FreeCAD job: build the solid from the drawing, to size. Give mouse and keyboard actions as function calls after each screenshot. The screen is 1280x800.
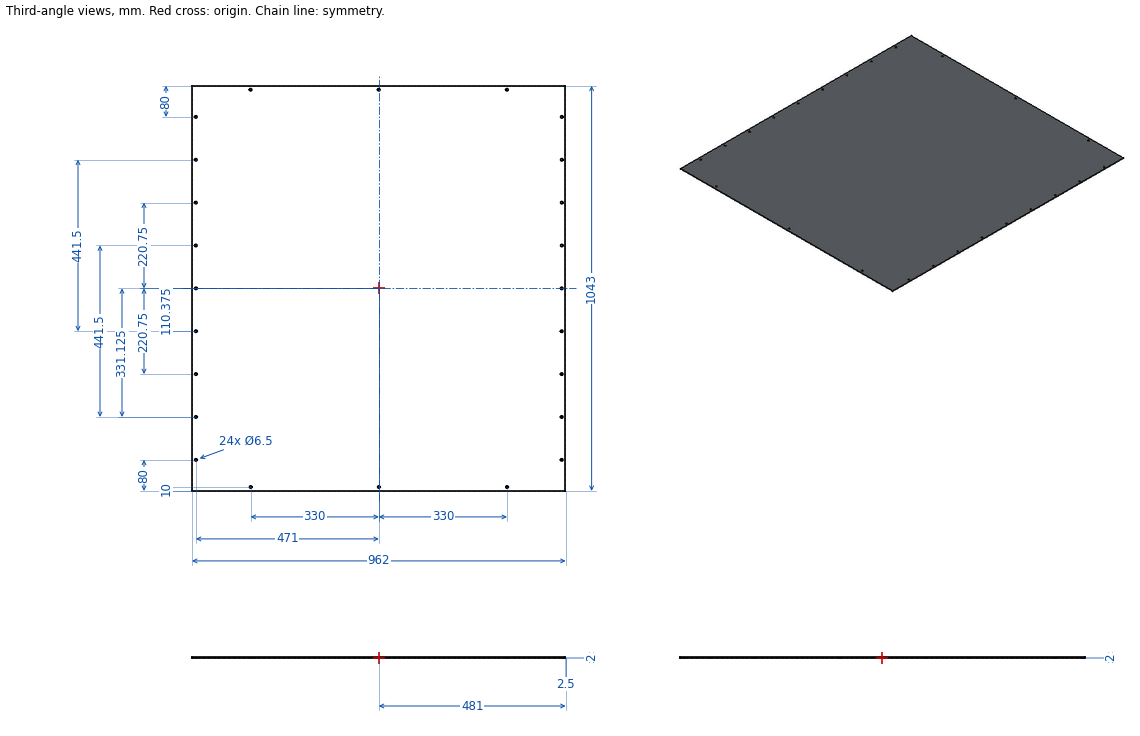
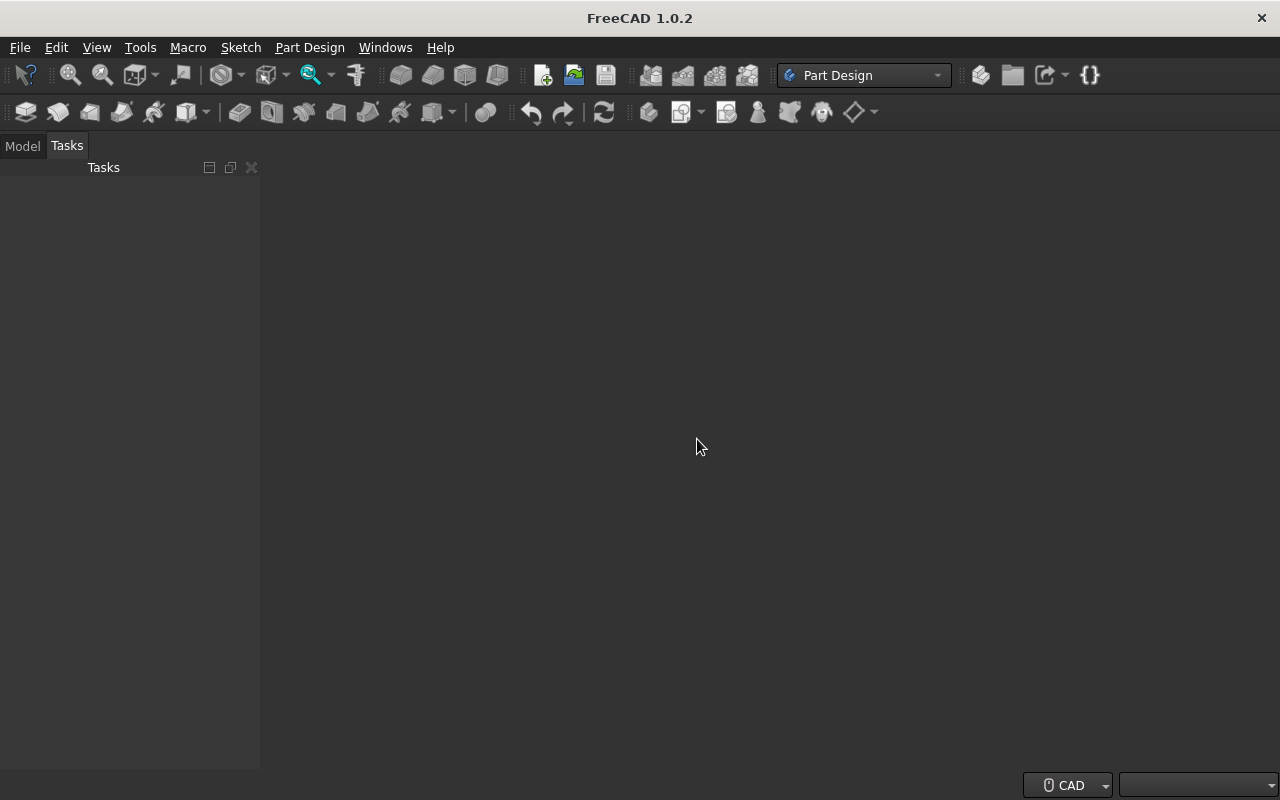
click(542, 76)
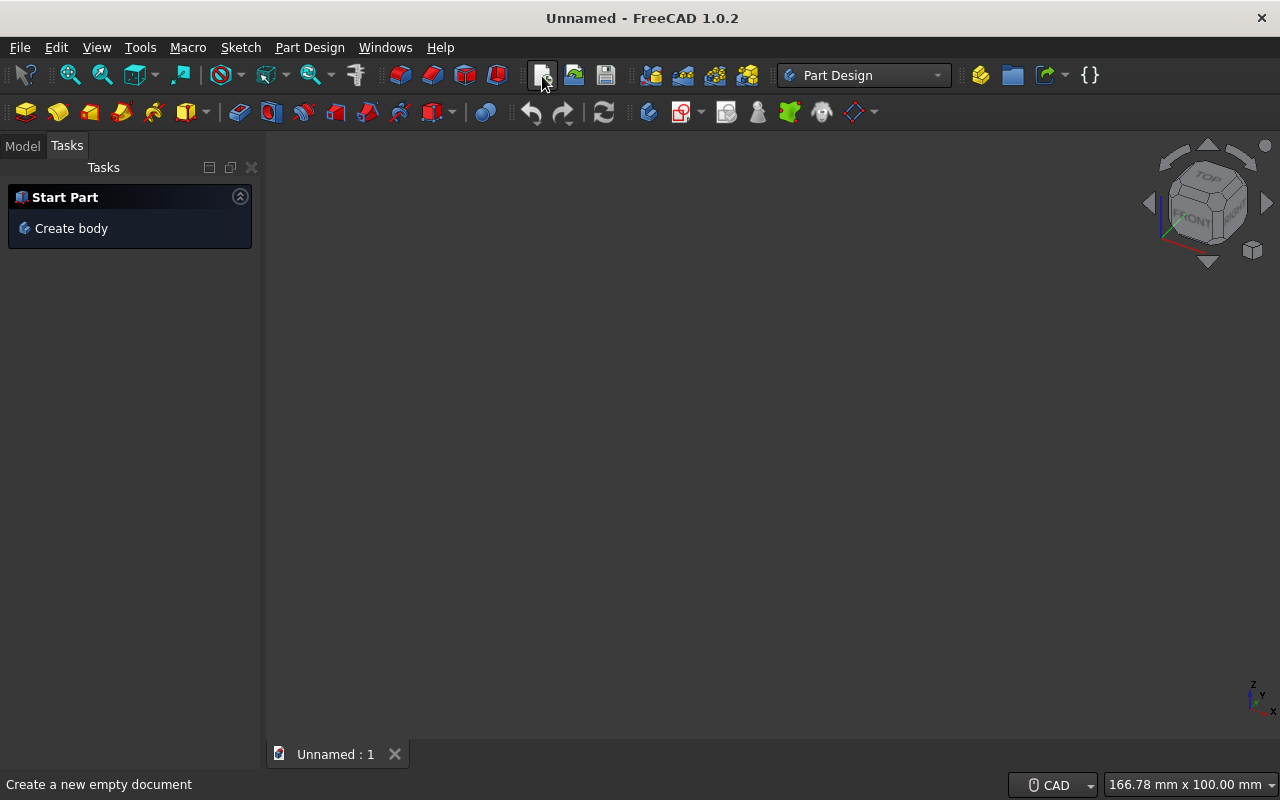
click(682, 112)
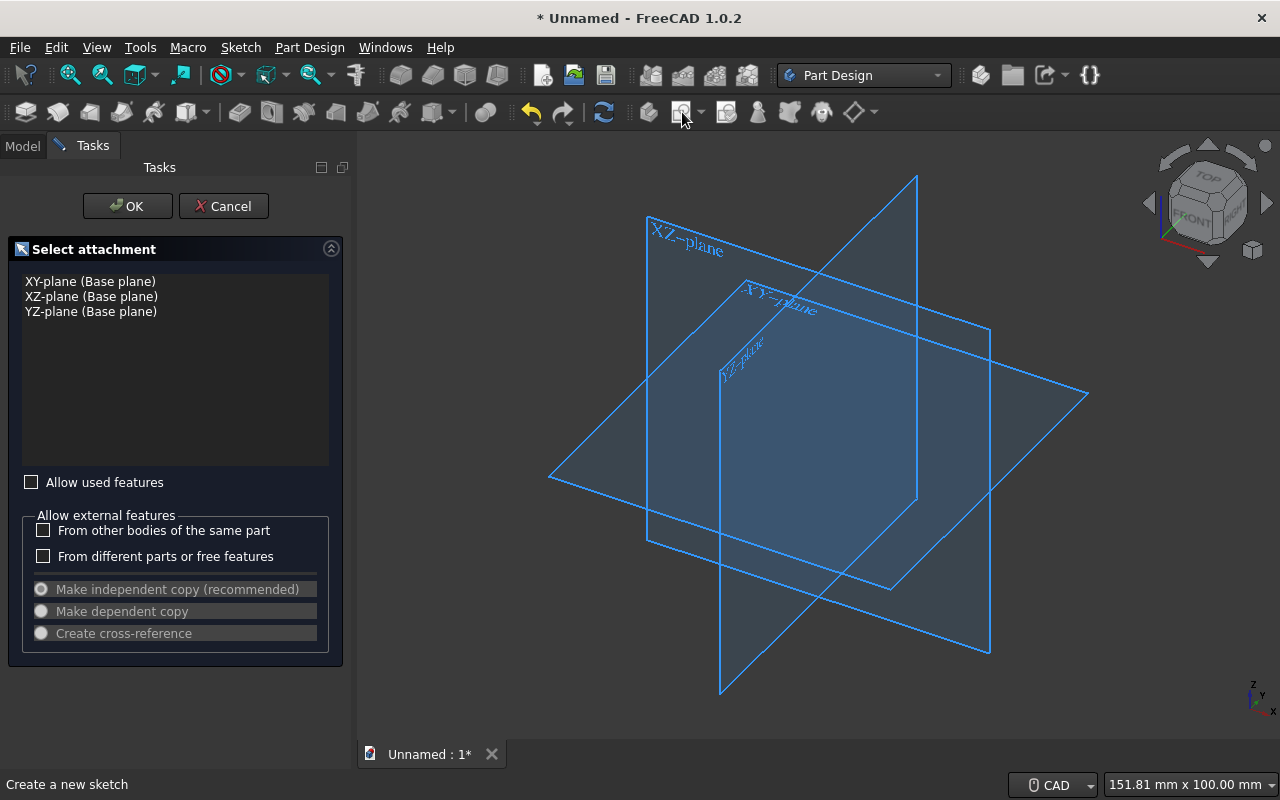
click(82, 282)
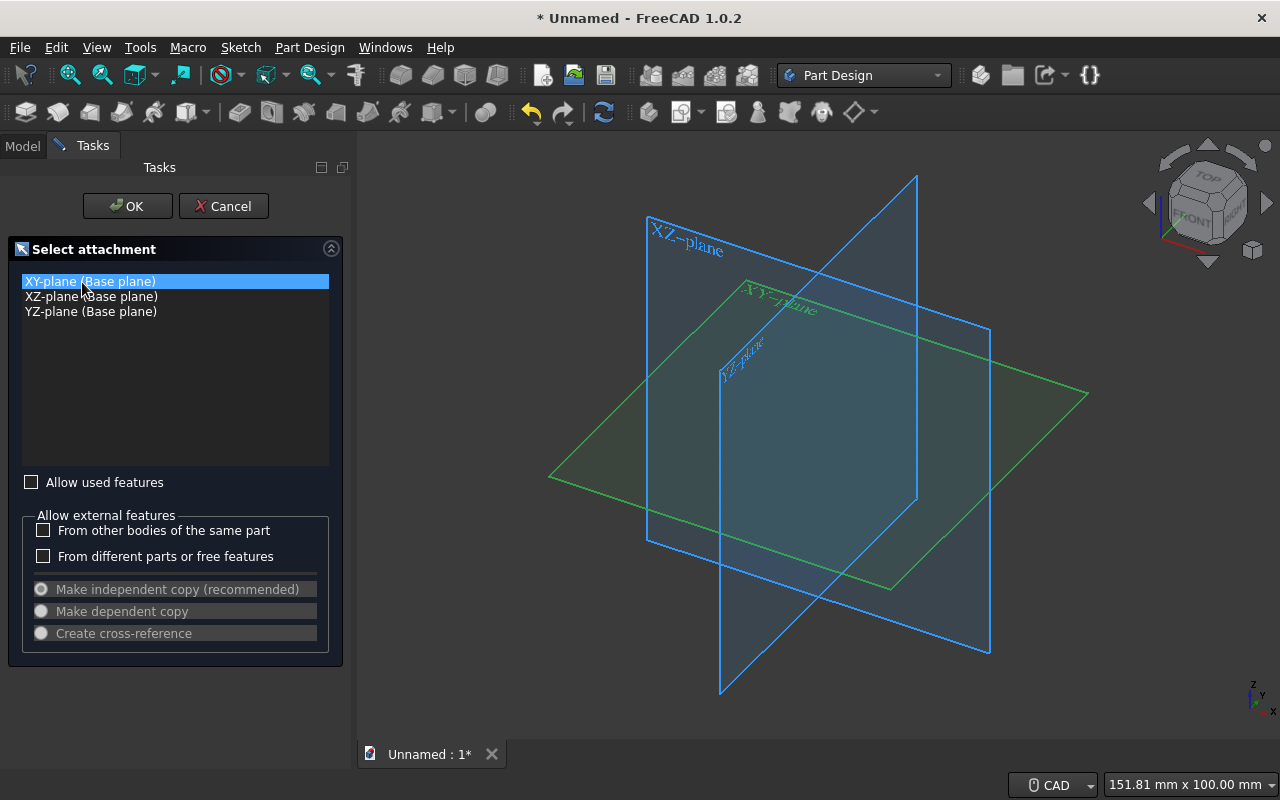
click(128, 206)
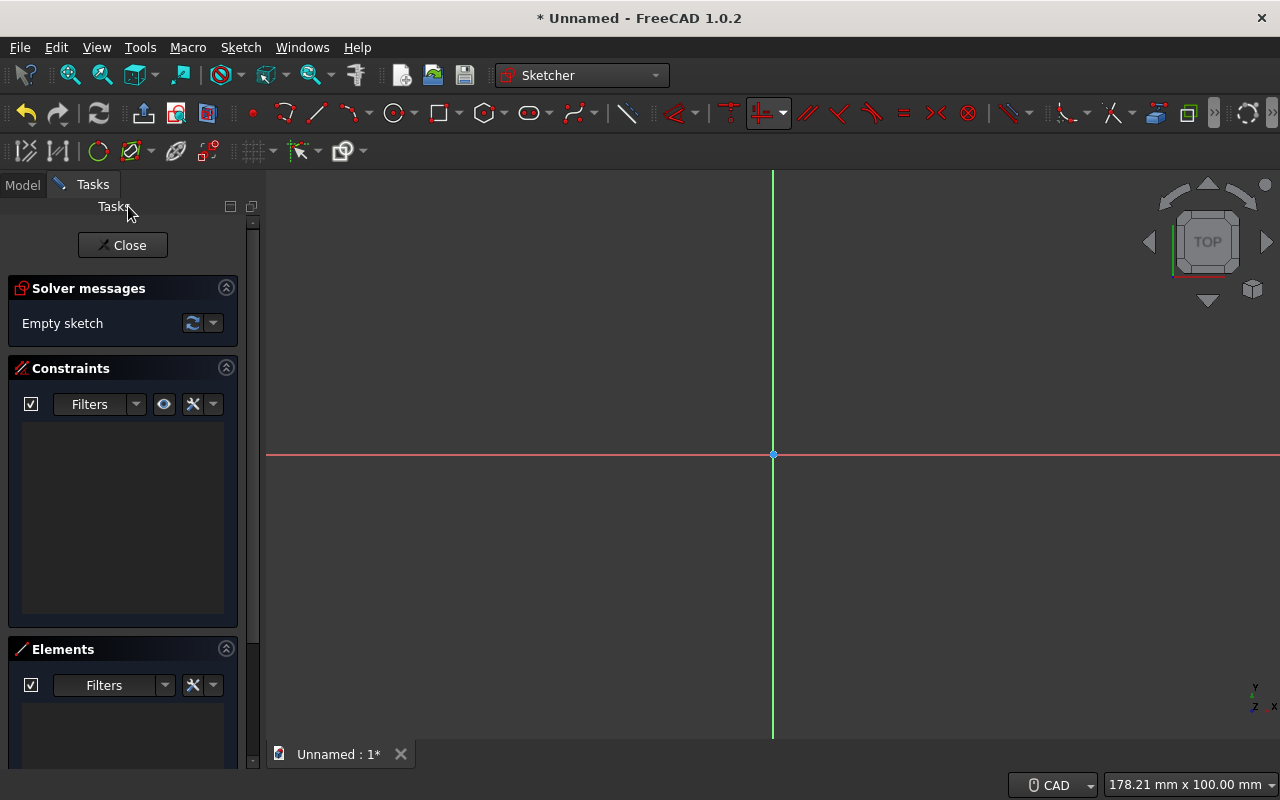
scroll(700, 454, down, 14)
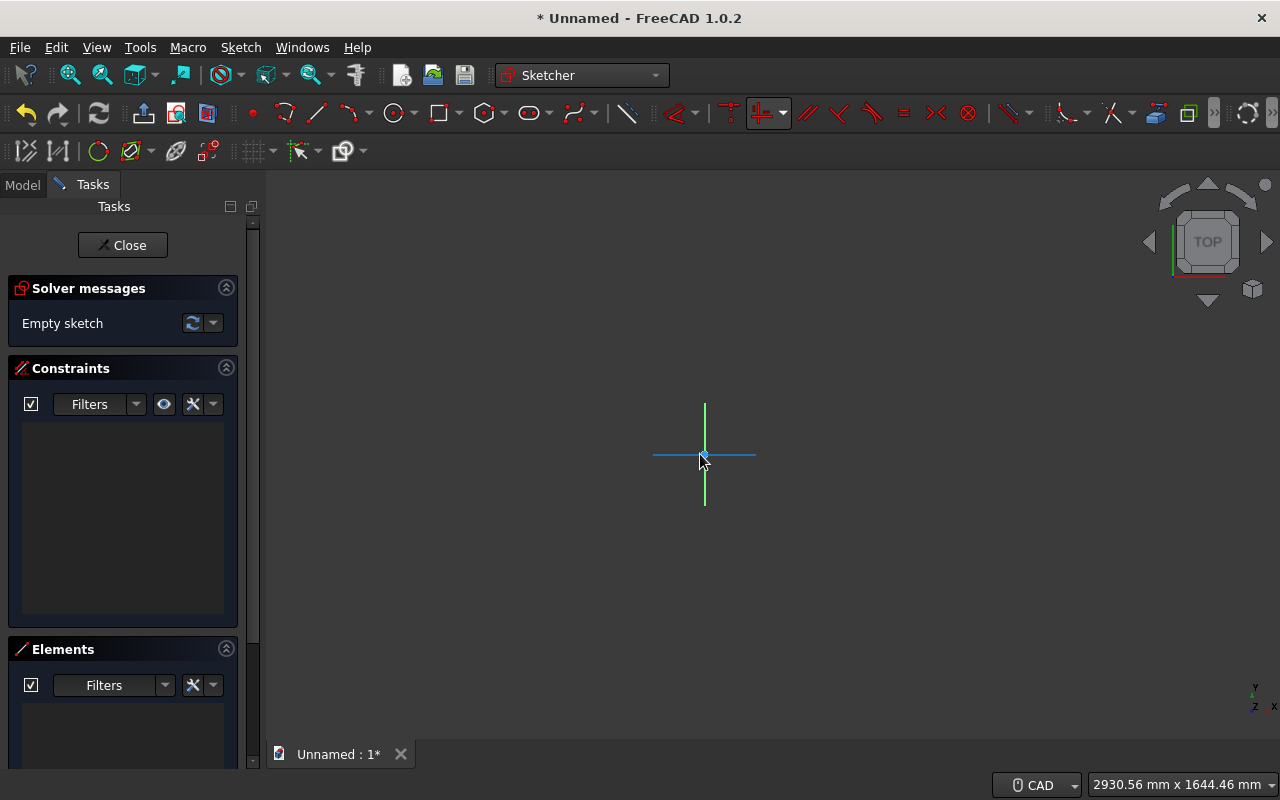
click(462, 114)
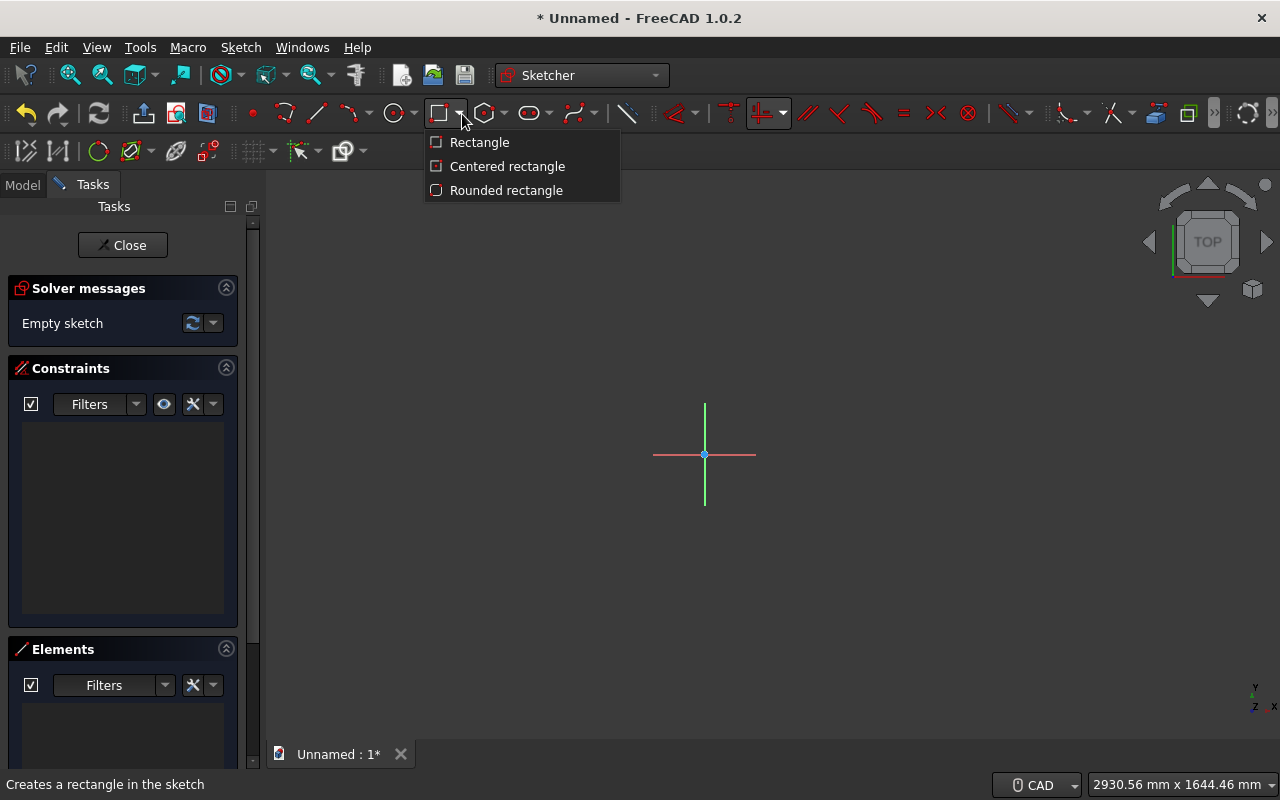
click(522, 166)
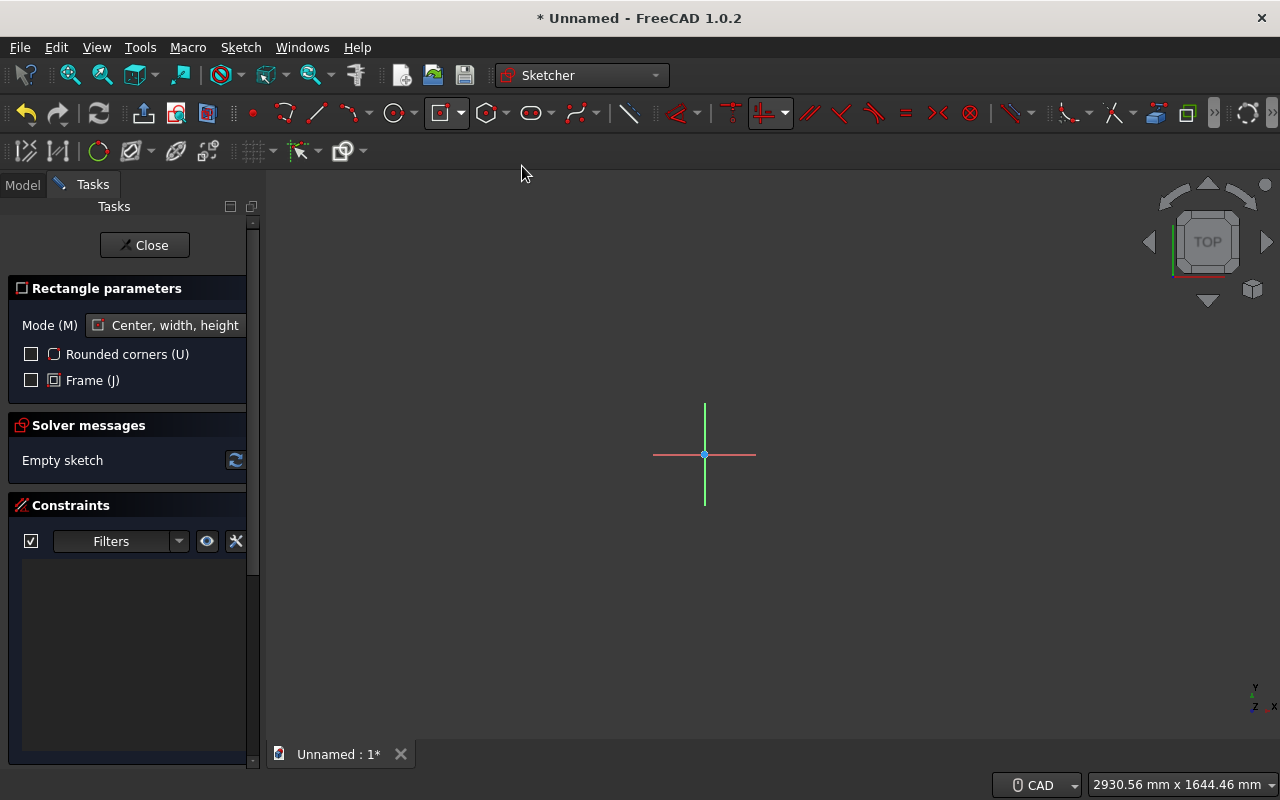
click(705, 454)
move(871, 274)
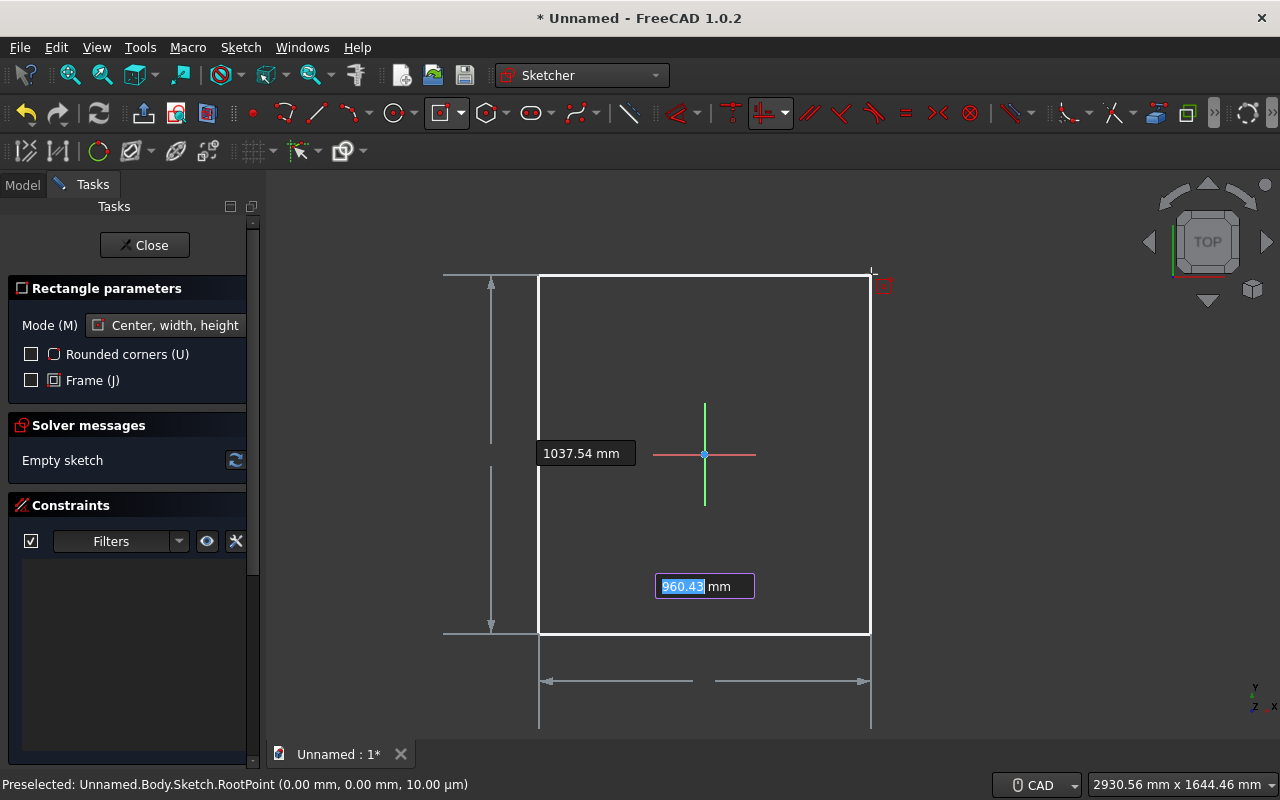
text(962)
key(Tab)
text(1043)
key(Return)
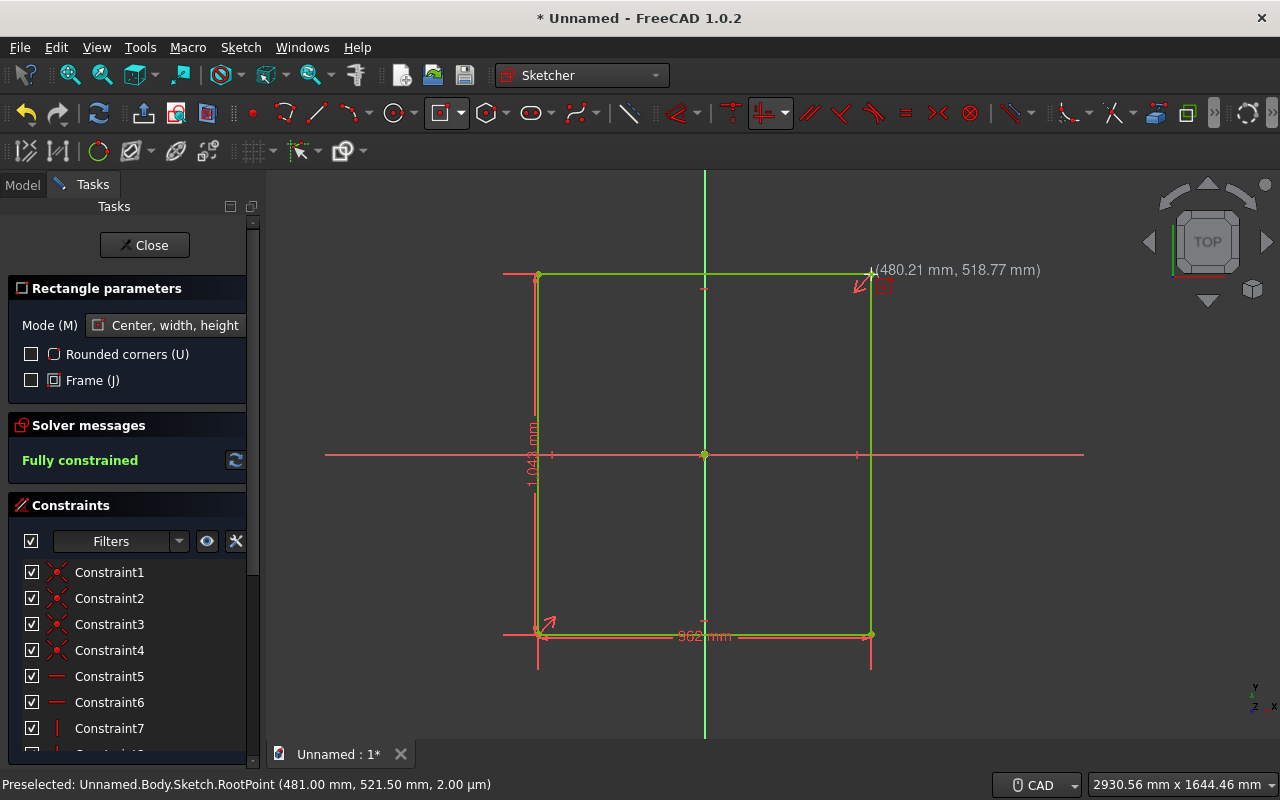
click(394, 114)